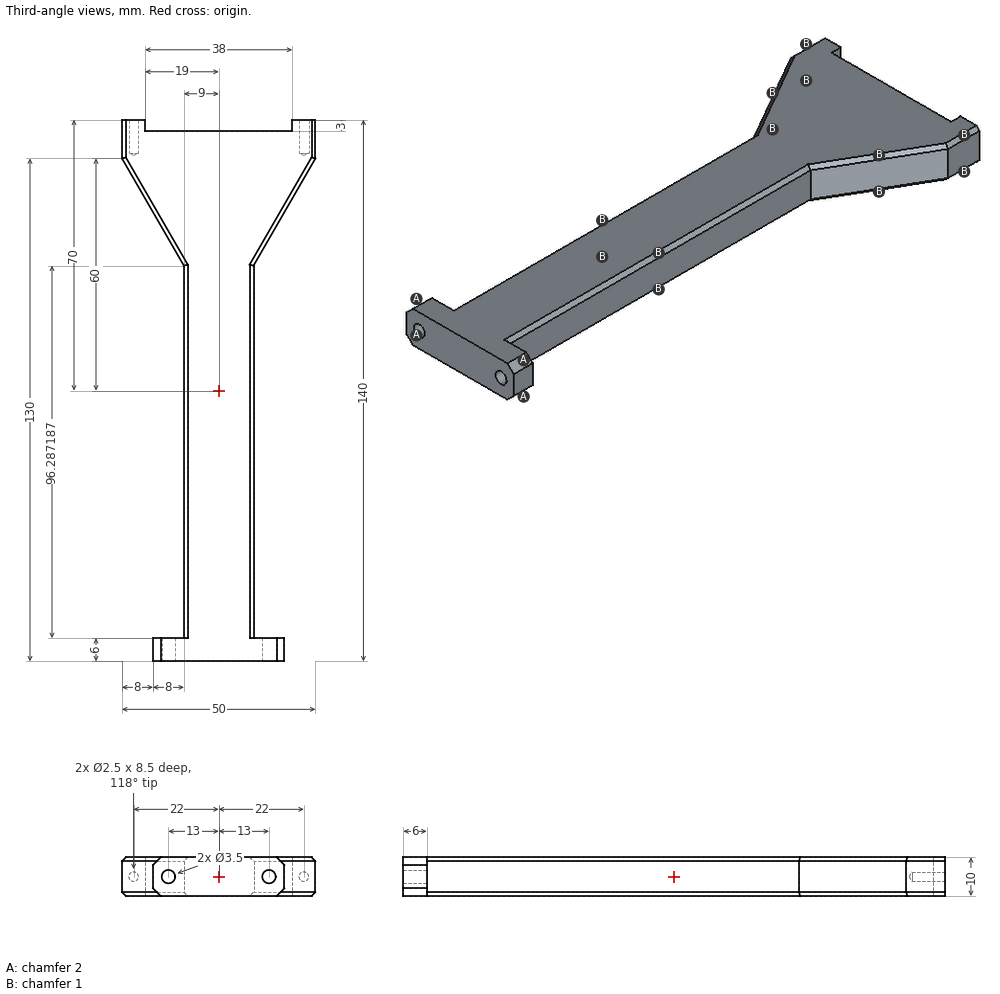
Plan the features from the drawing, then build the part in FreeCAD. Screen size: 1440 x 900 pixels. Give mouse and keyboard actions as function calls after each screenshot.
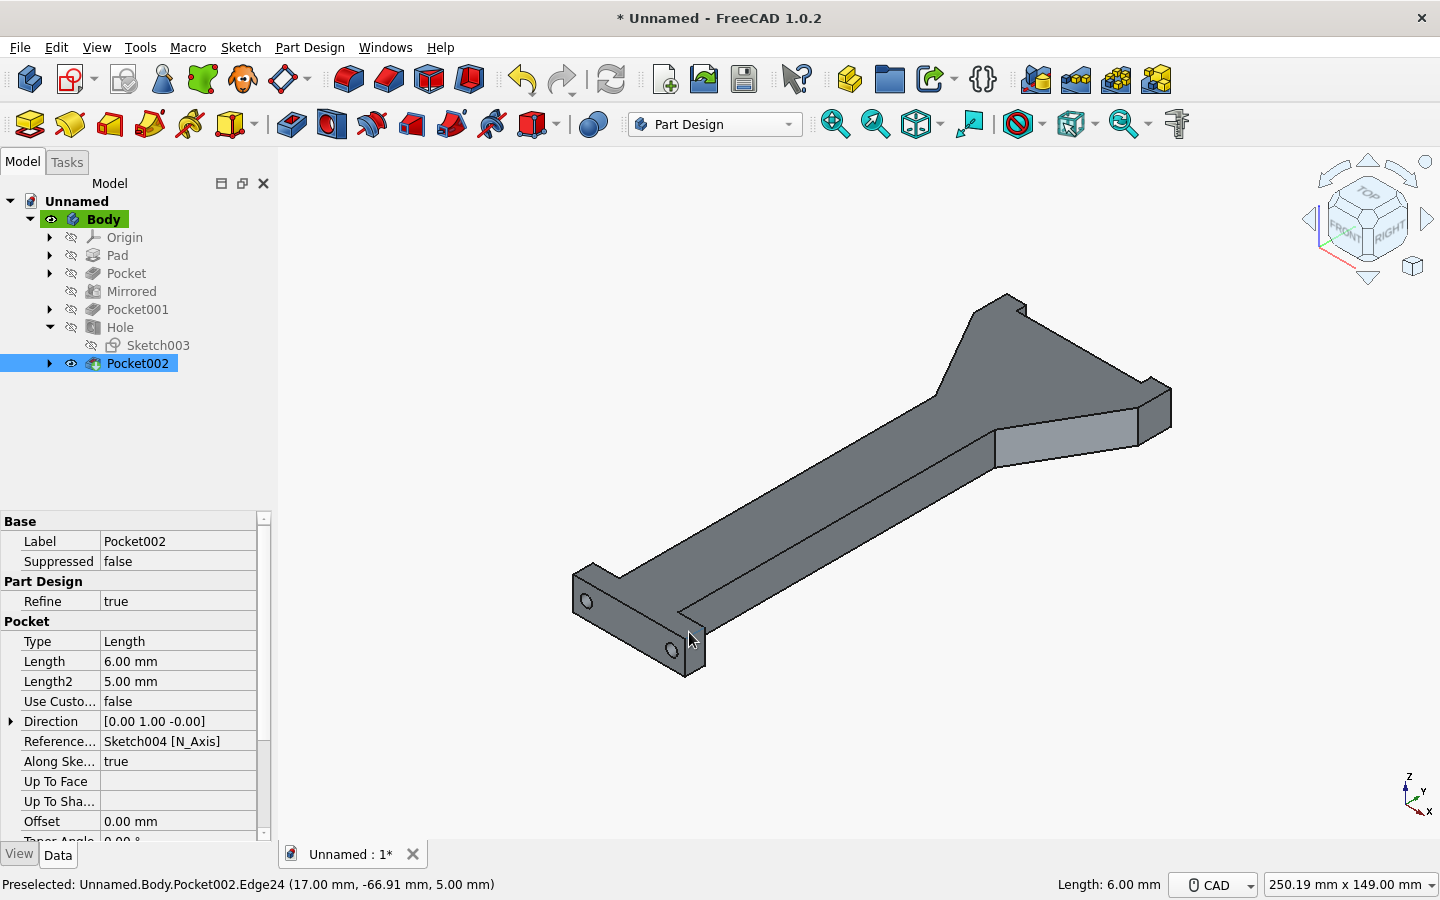
key(2)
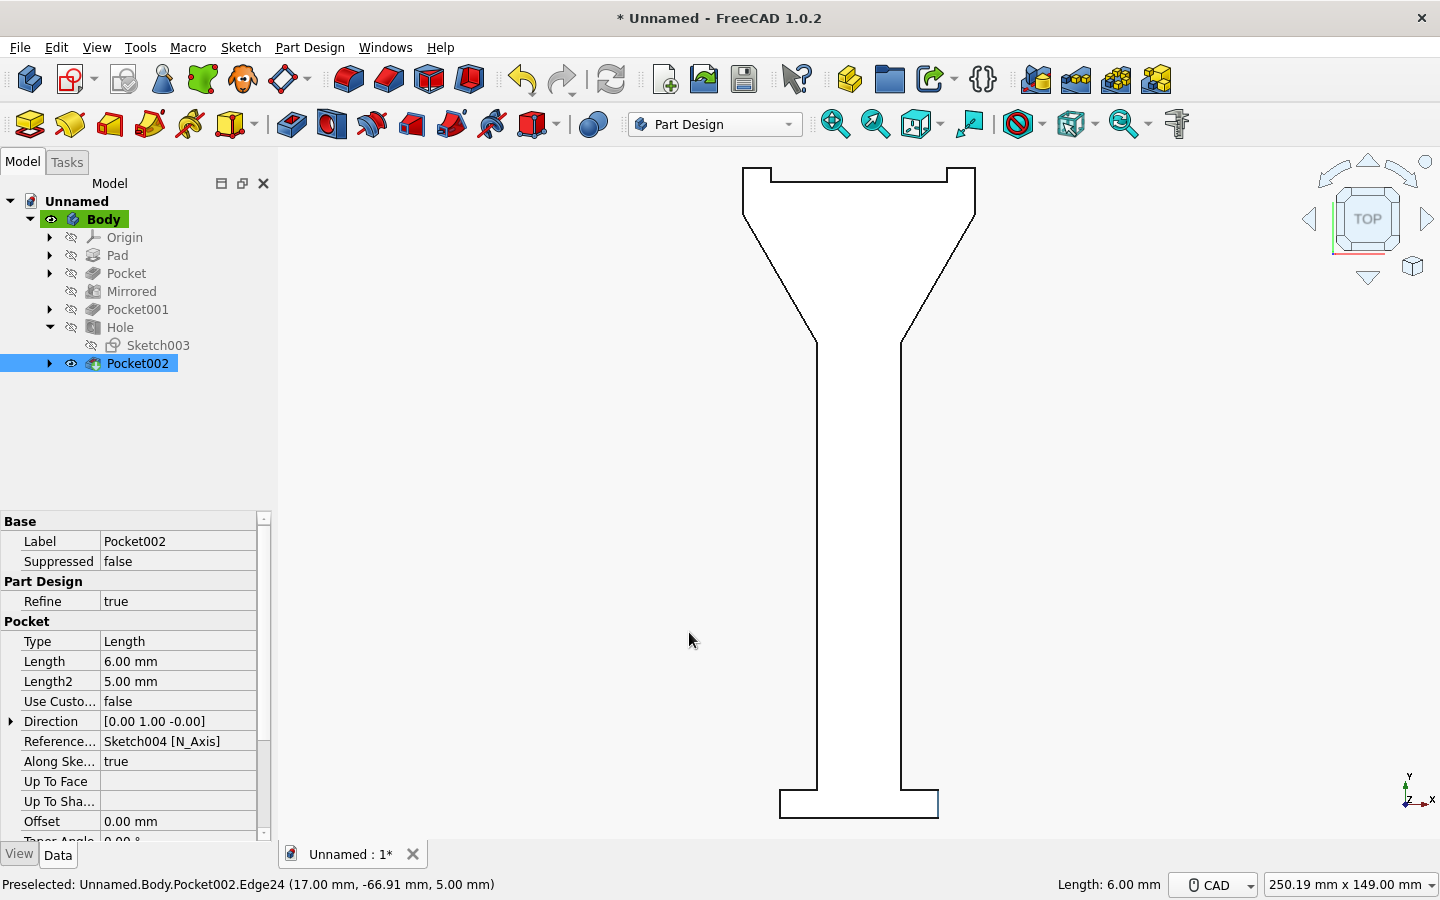
click(780, 803, ctrl)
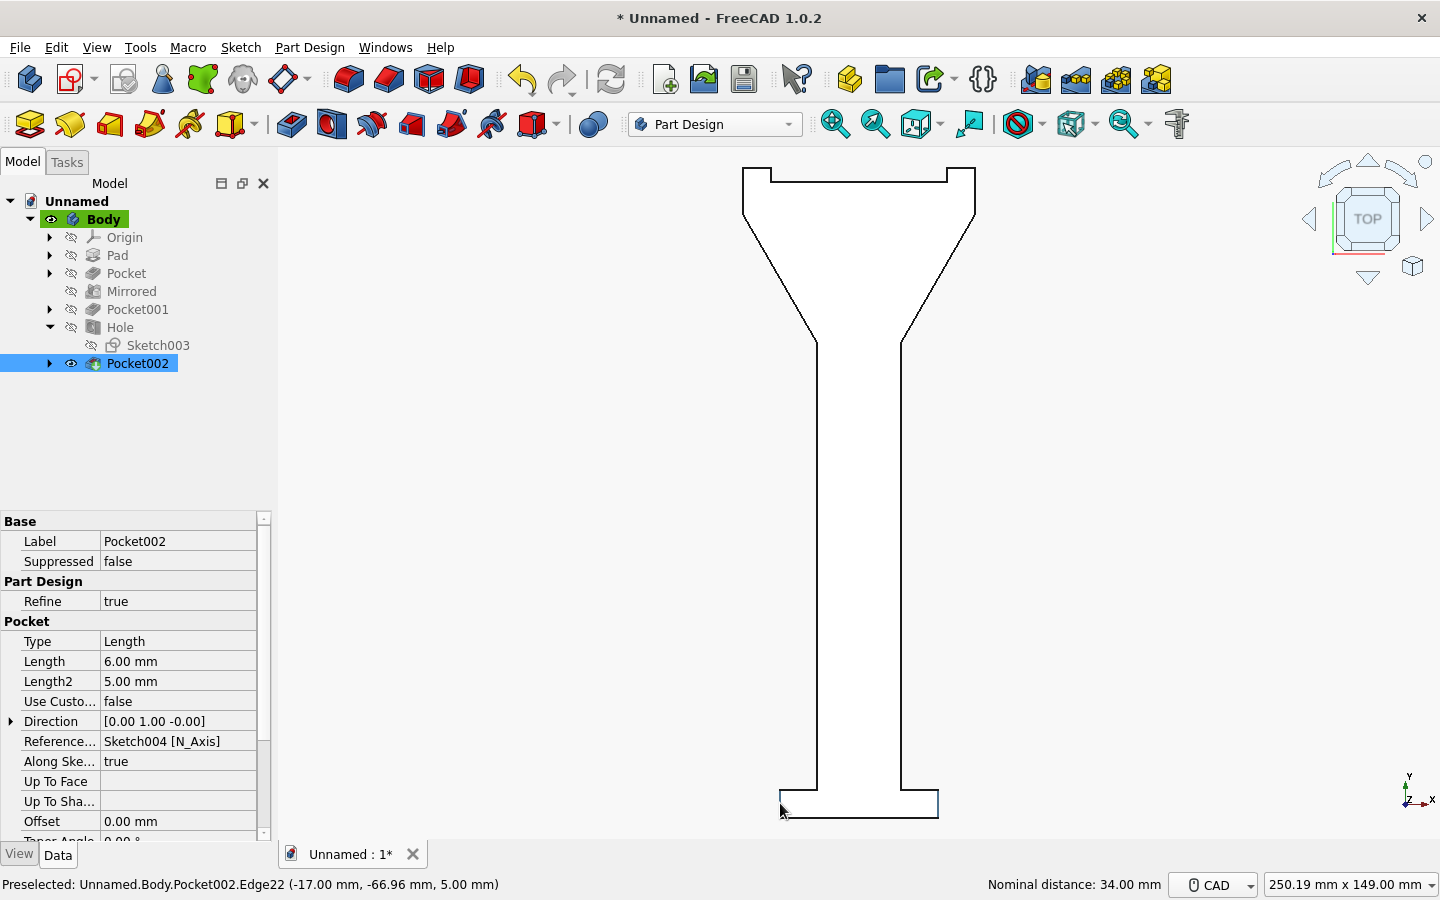
key(0)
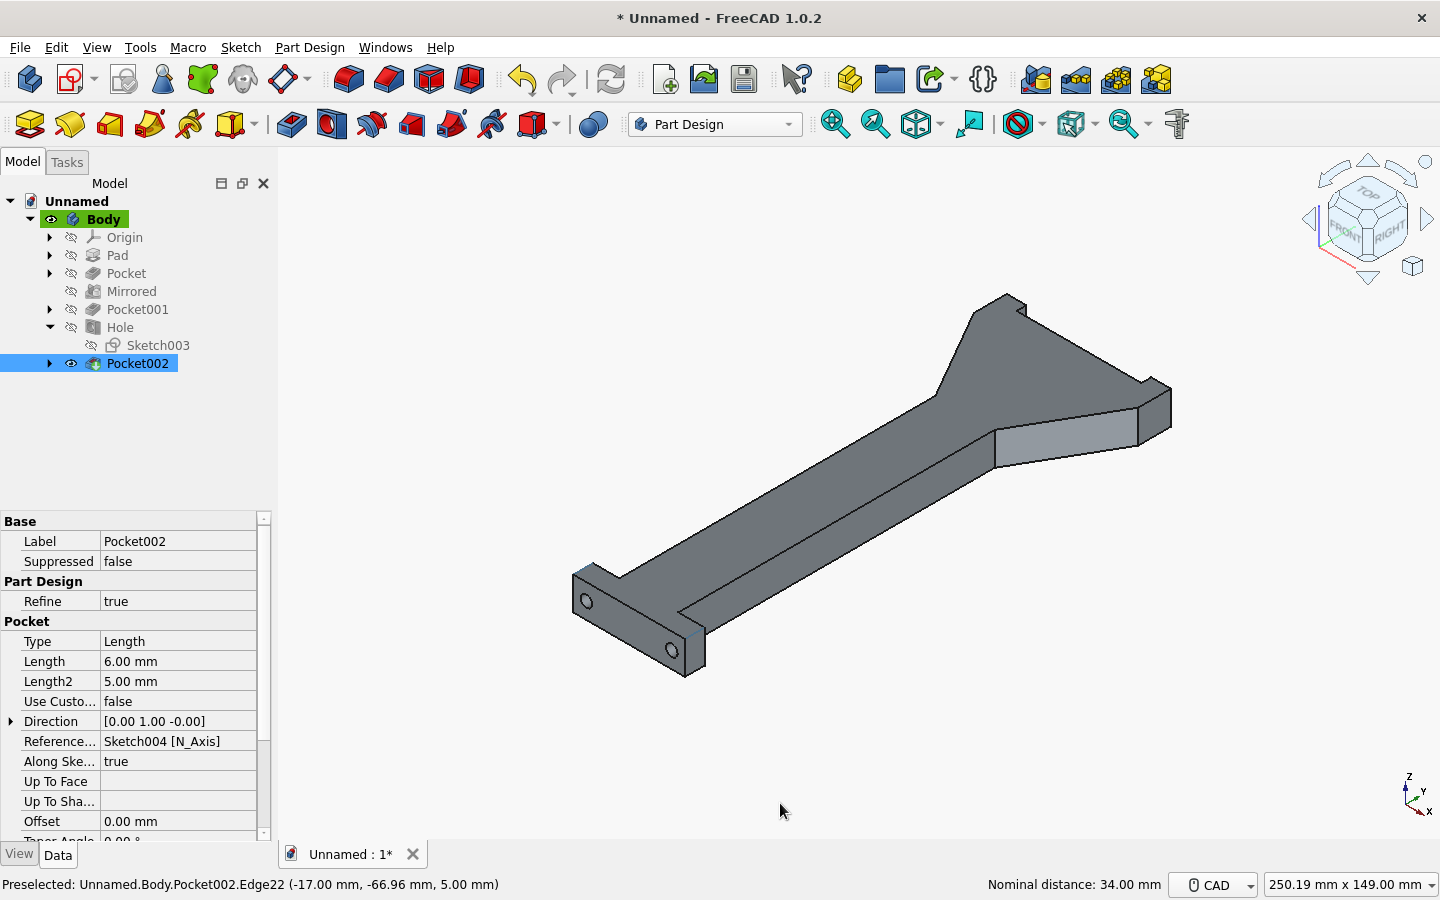
key(1)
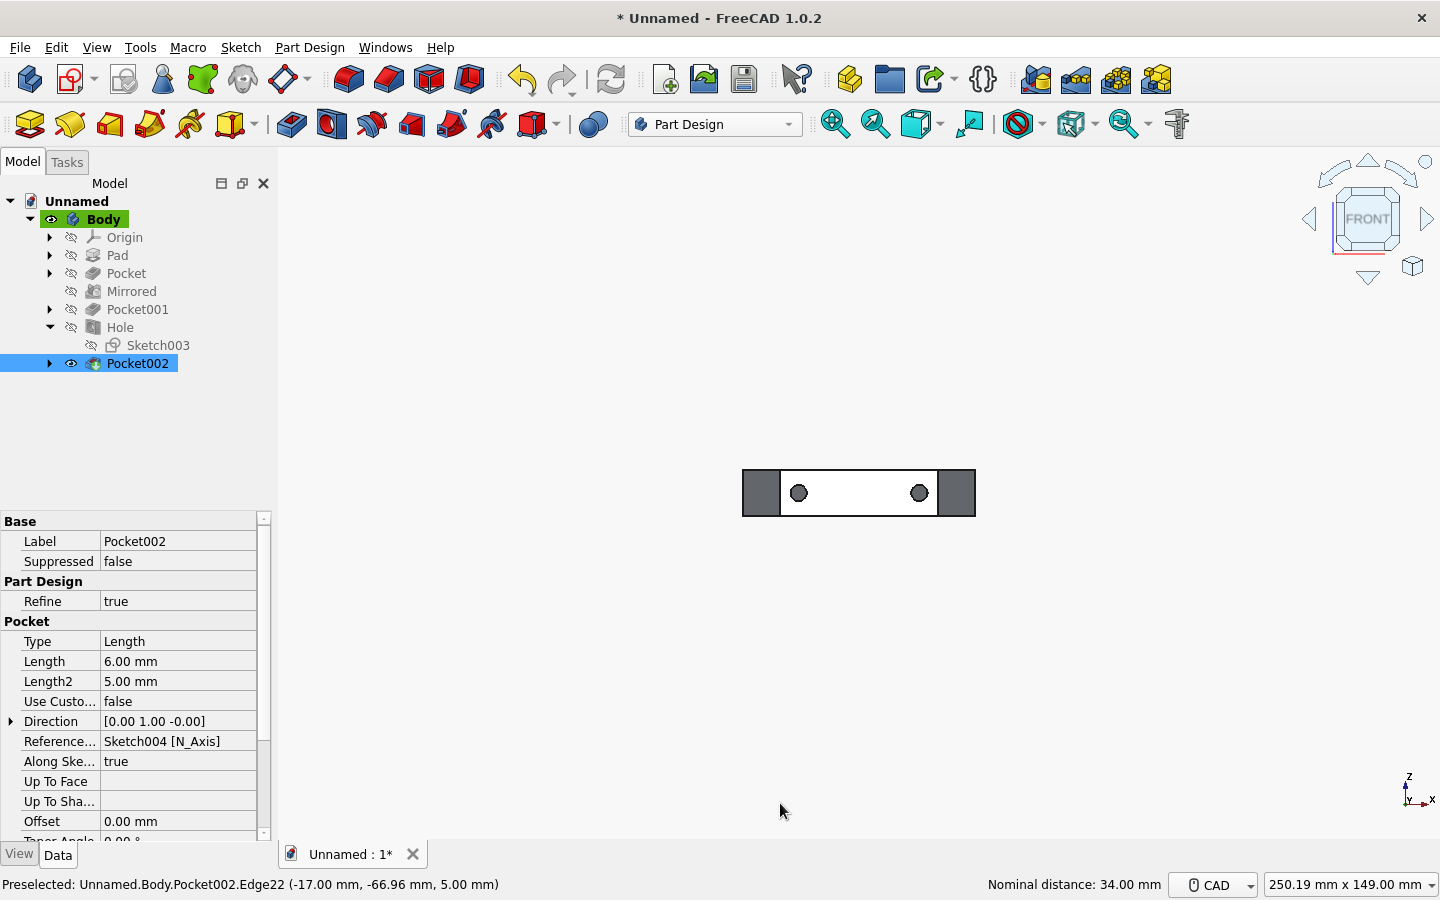
click(836, 124)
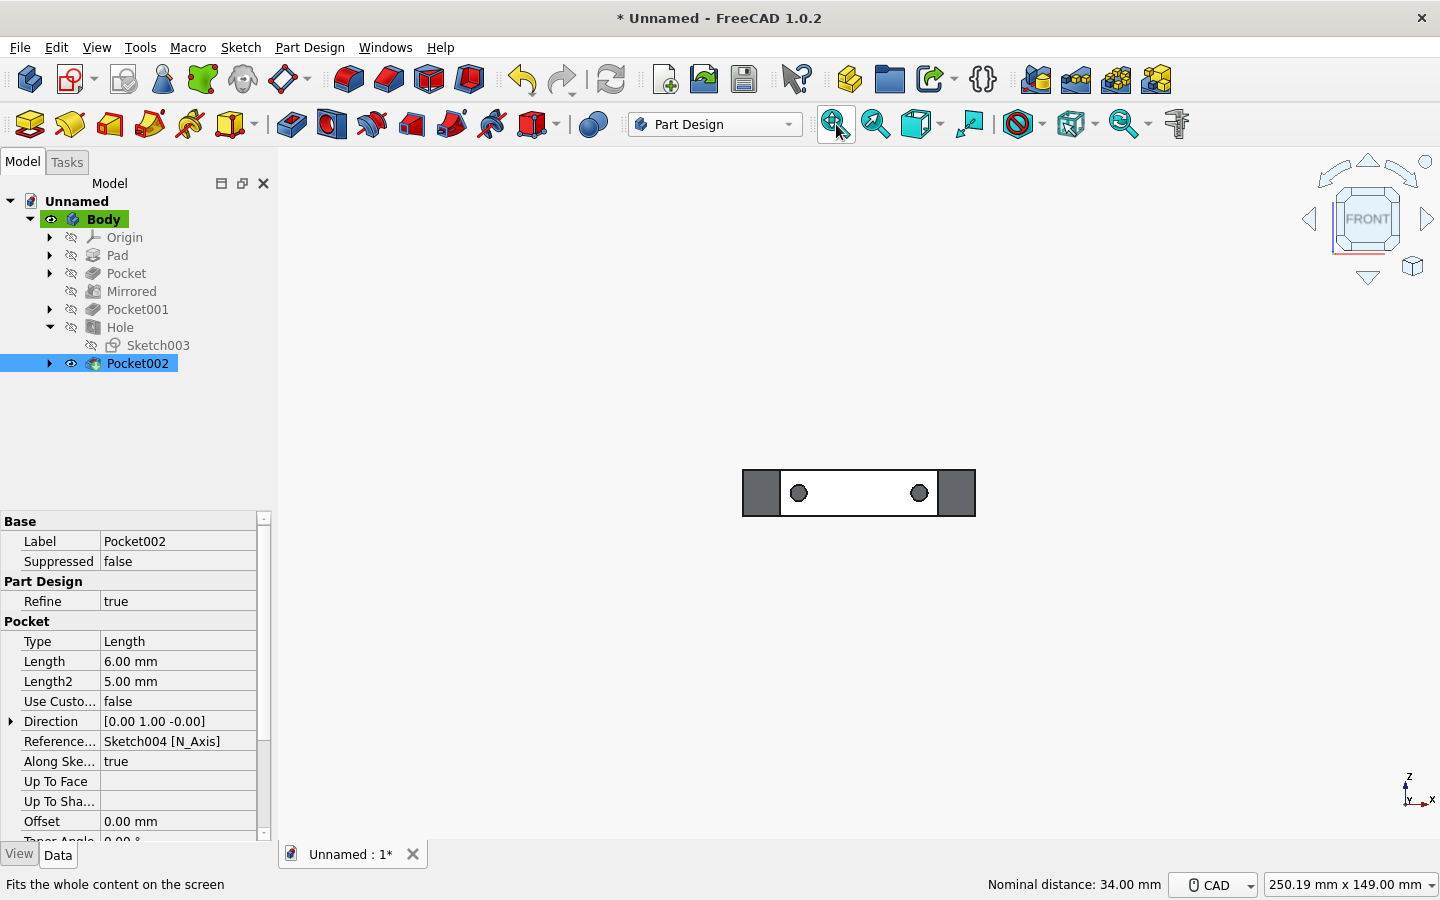
key(3)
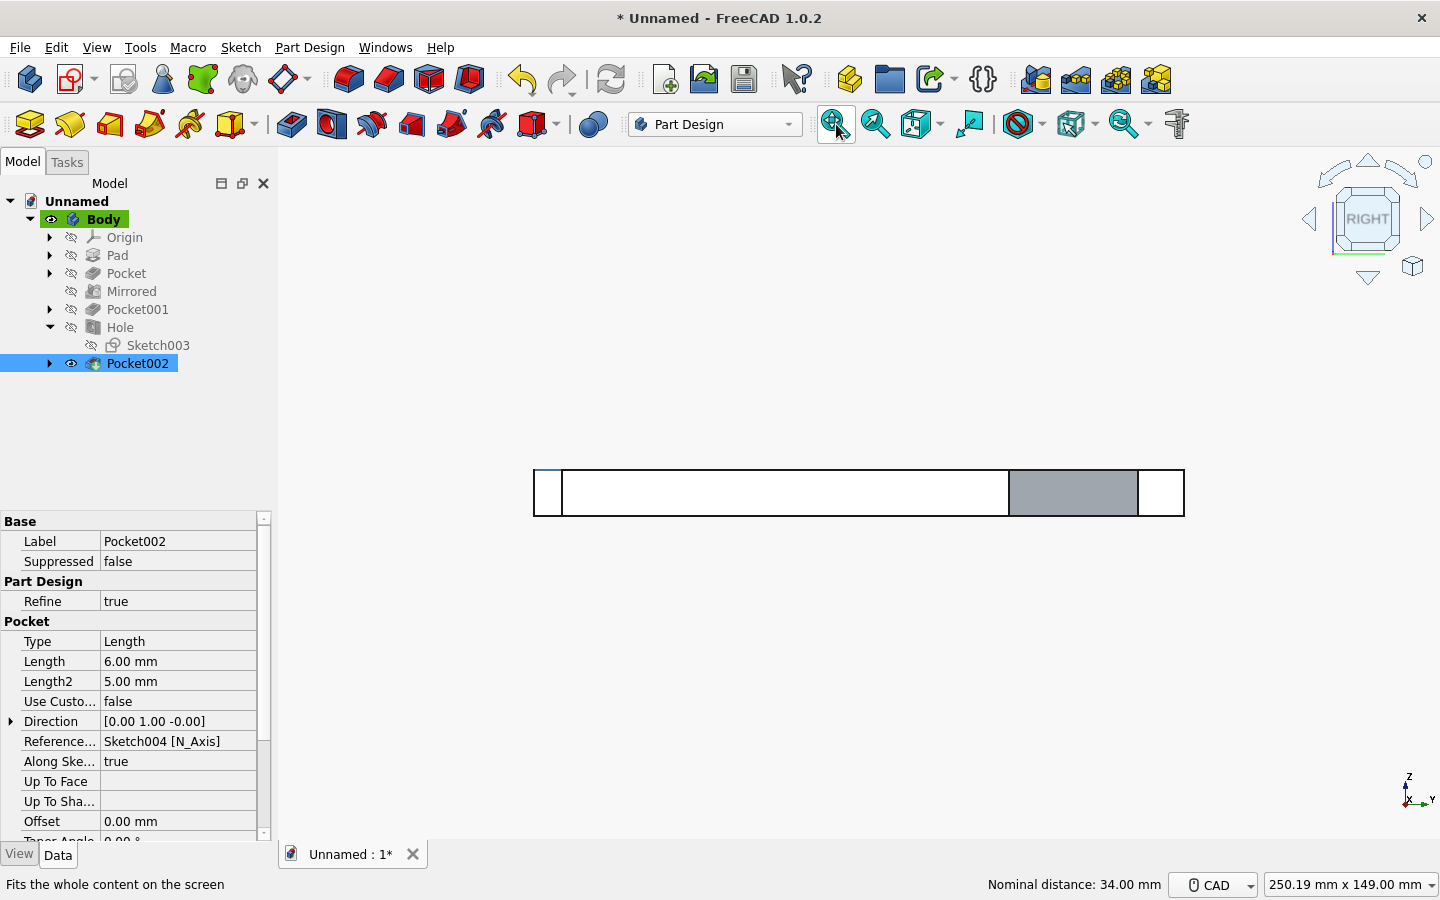
click(548, 515, ctrl)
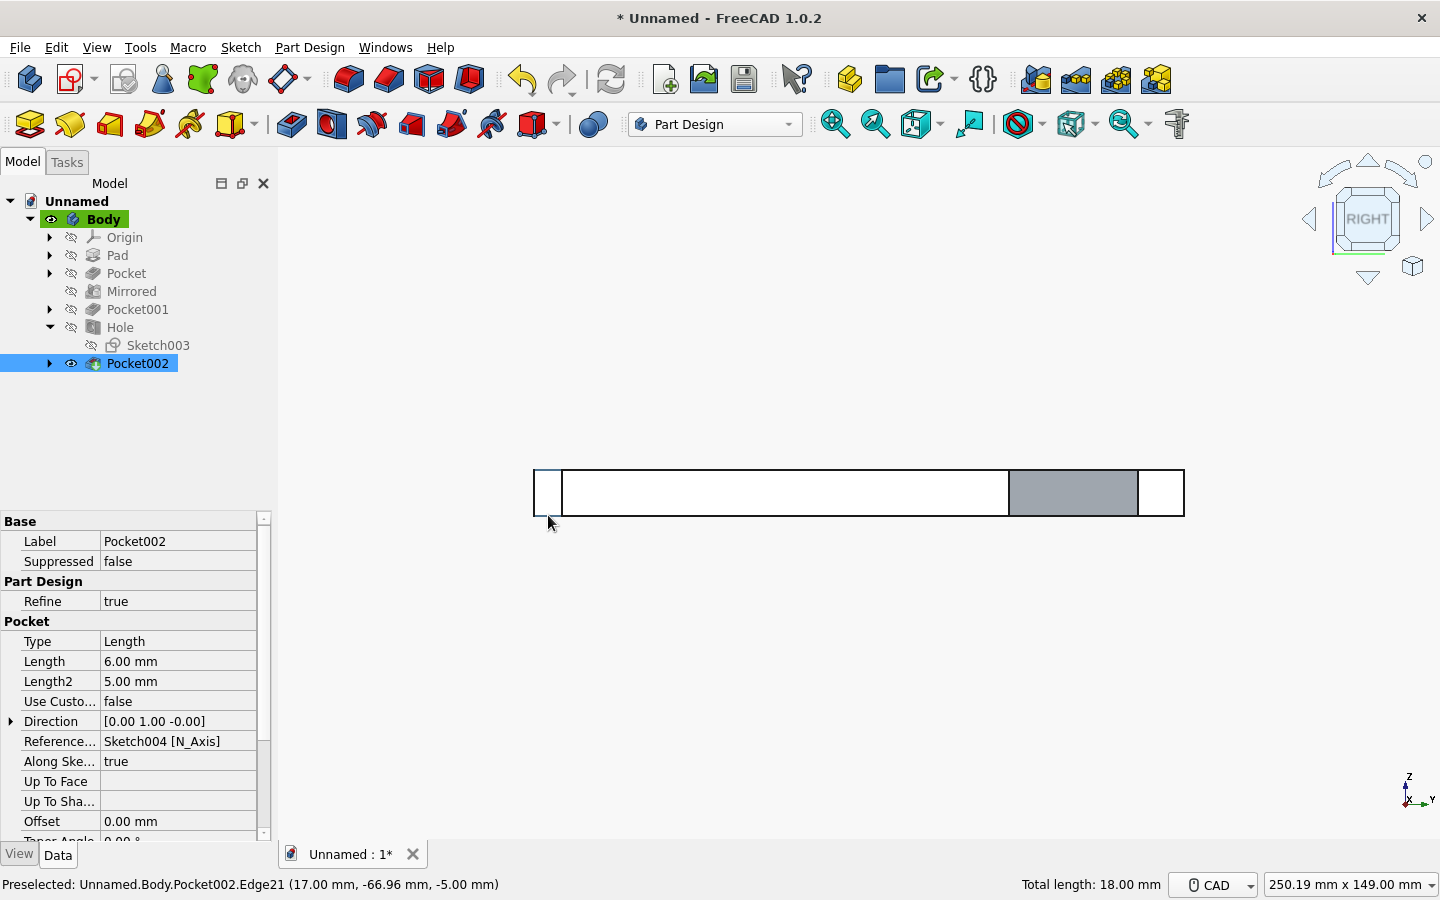
key(5)